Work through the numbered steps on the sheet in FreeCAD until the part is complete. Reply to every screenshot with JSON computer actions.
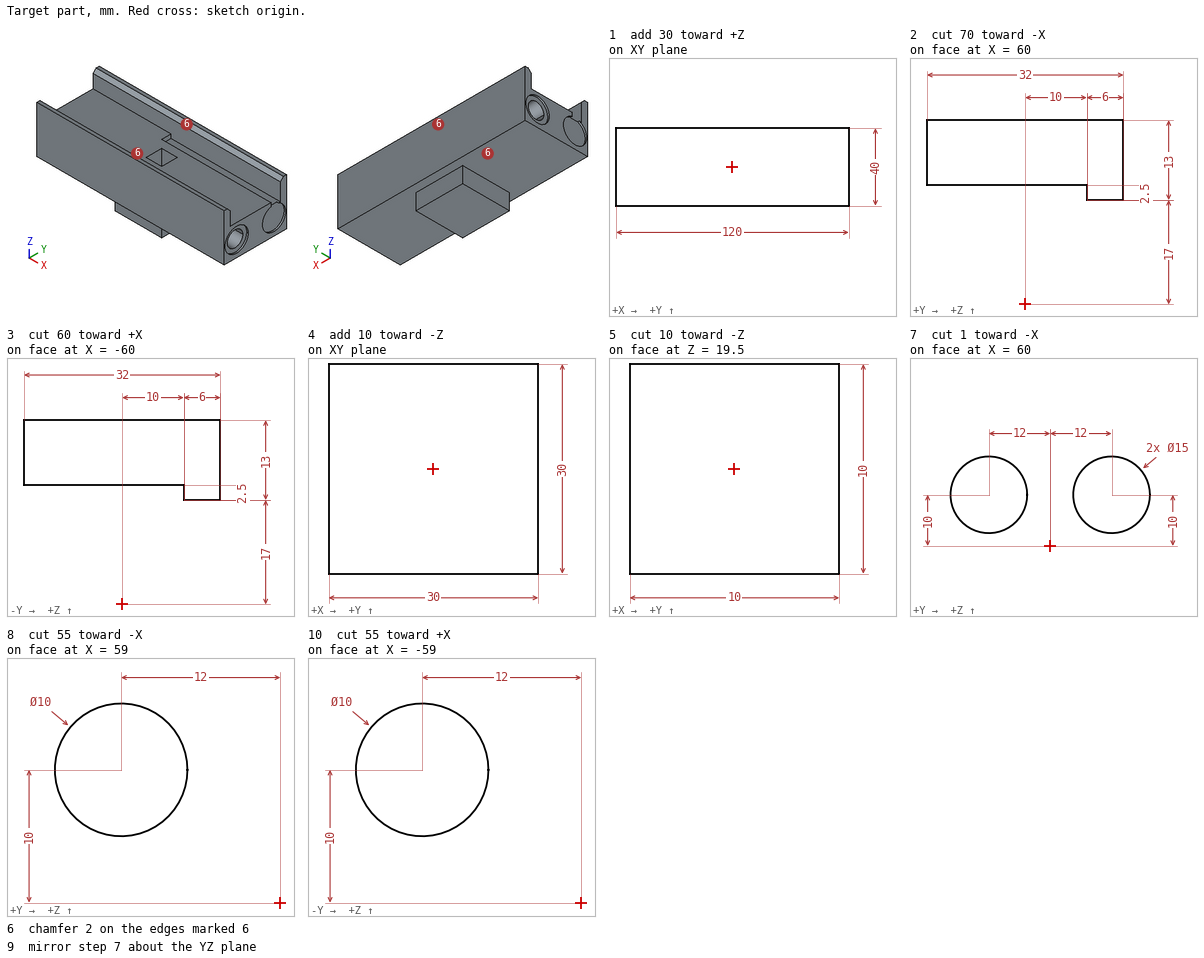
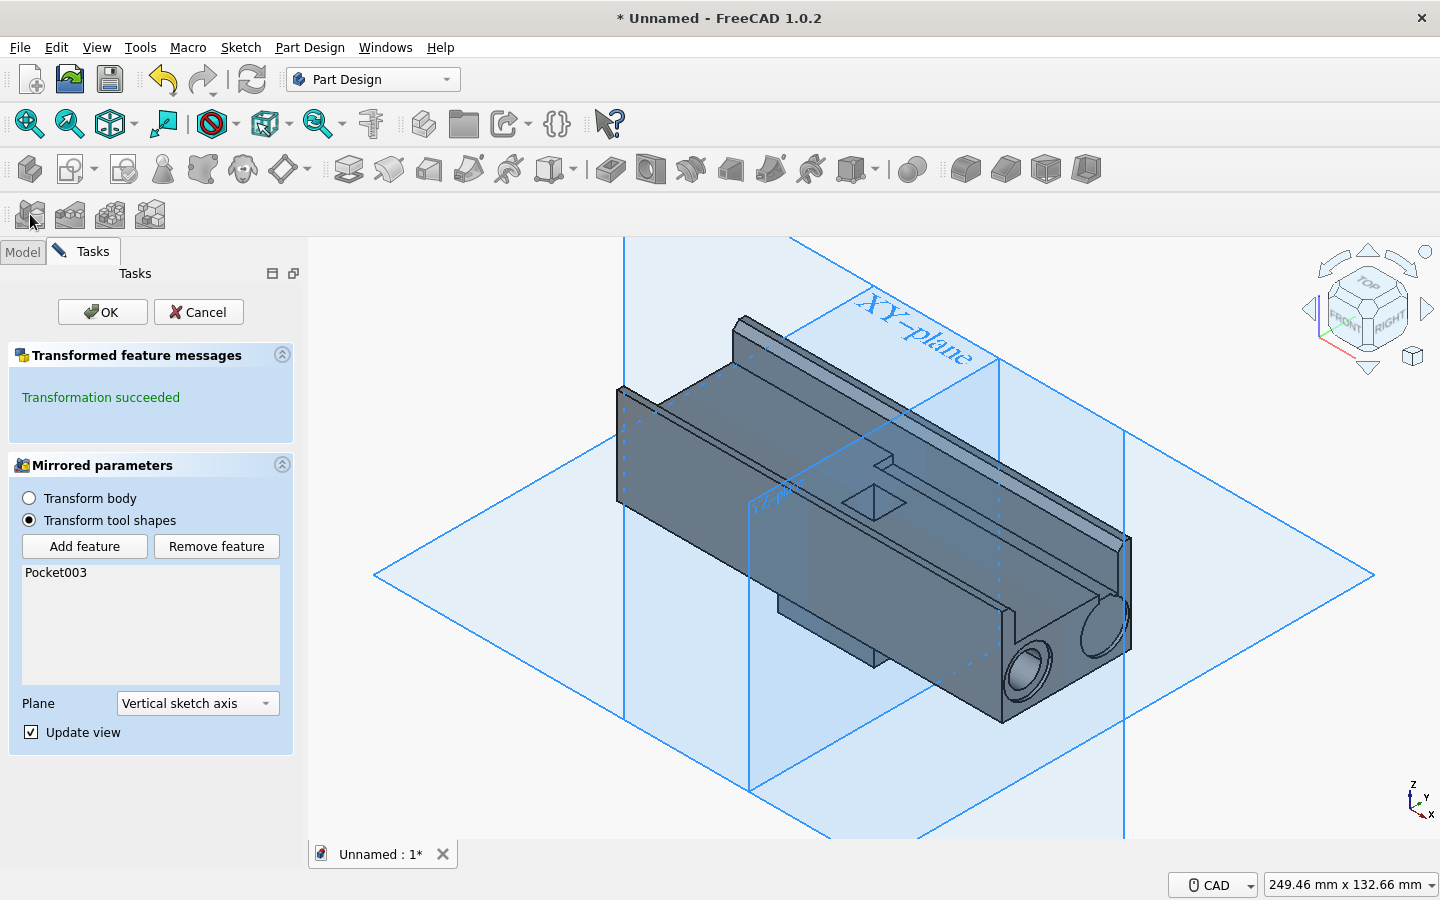
{"action": "left_click", "coordinate": [198, 704]}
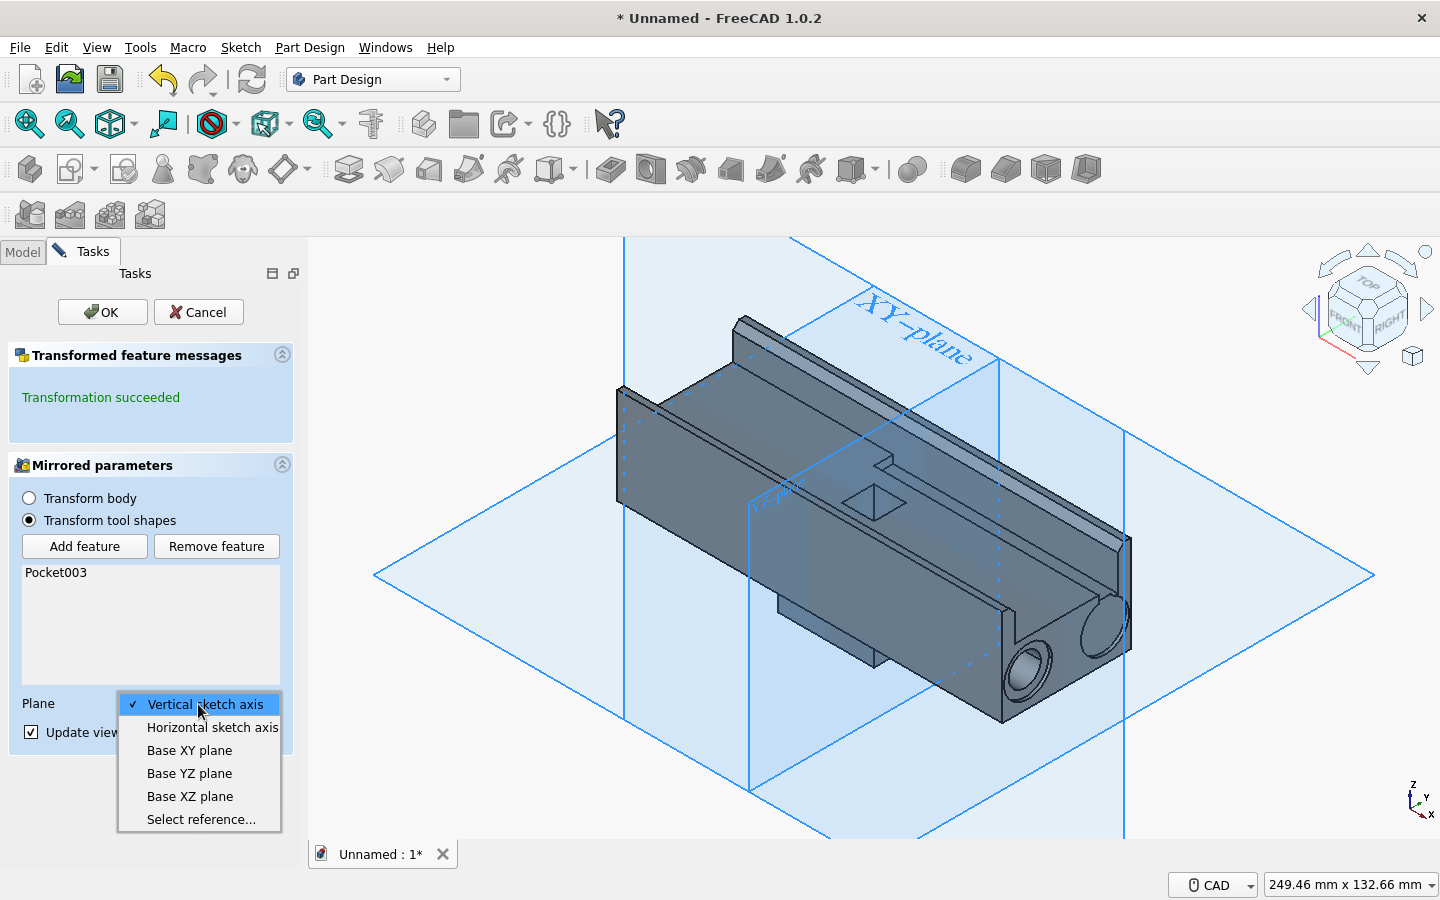
{"action": "left_click", "coordinate": [198, 774]}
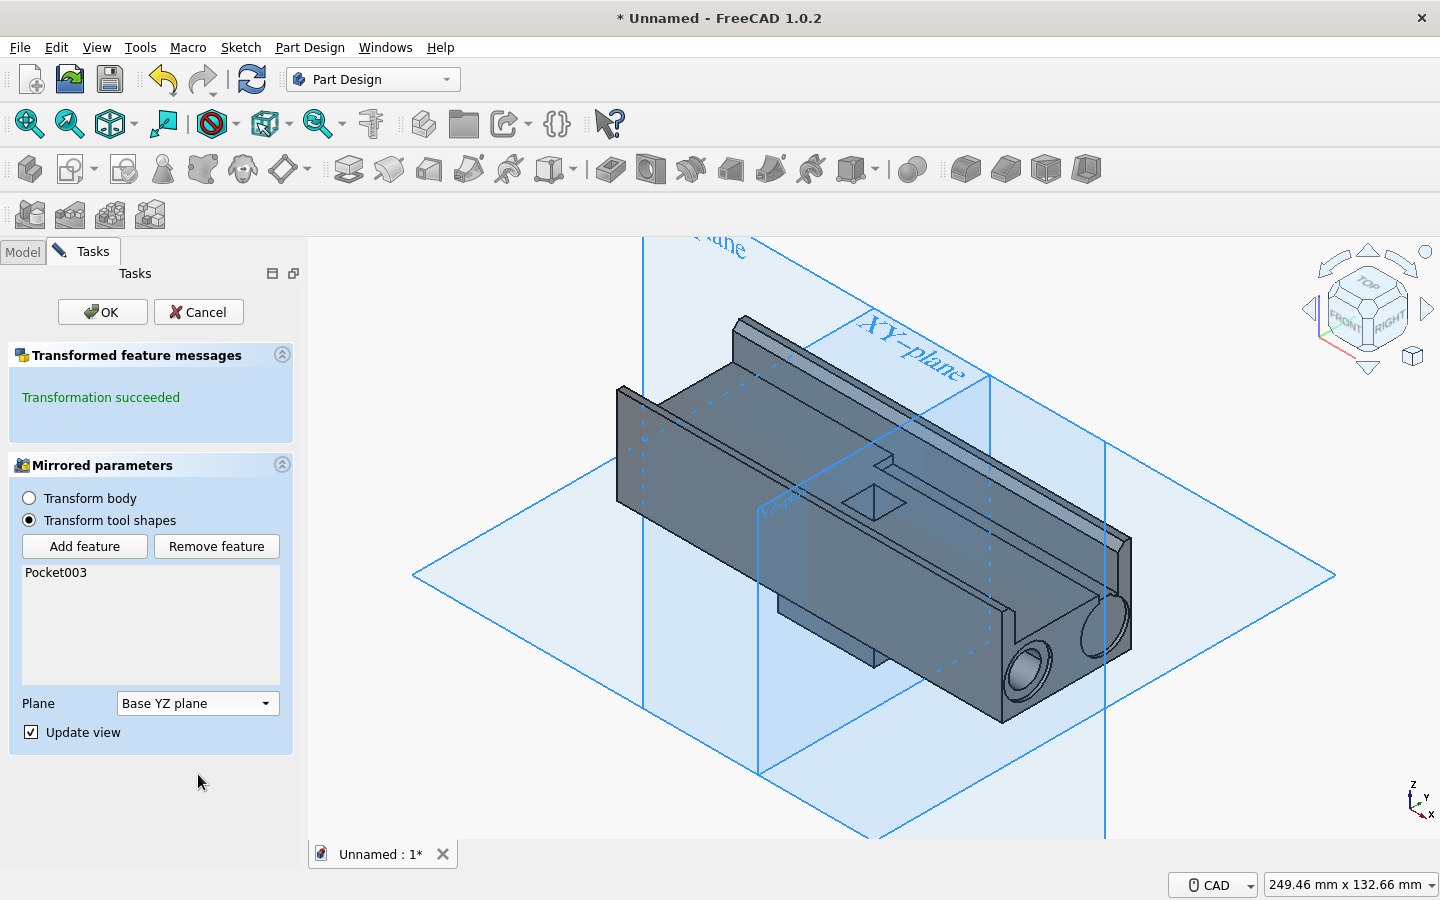
{"action": "left_click", "coordinate": [103, 312]}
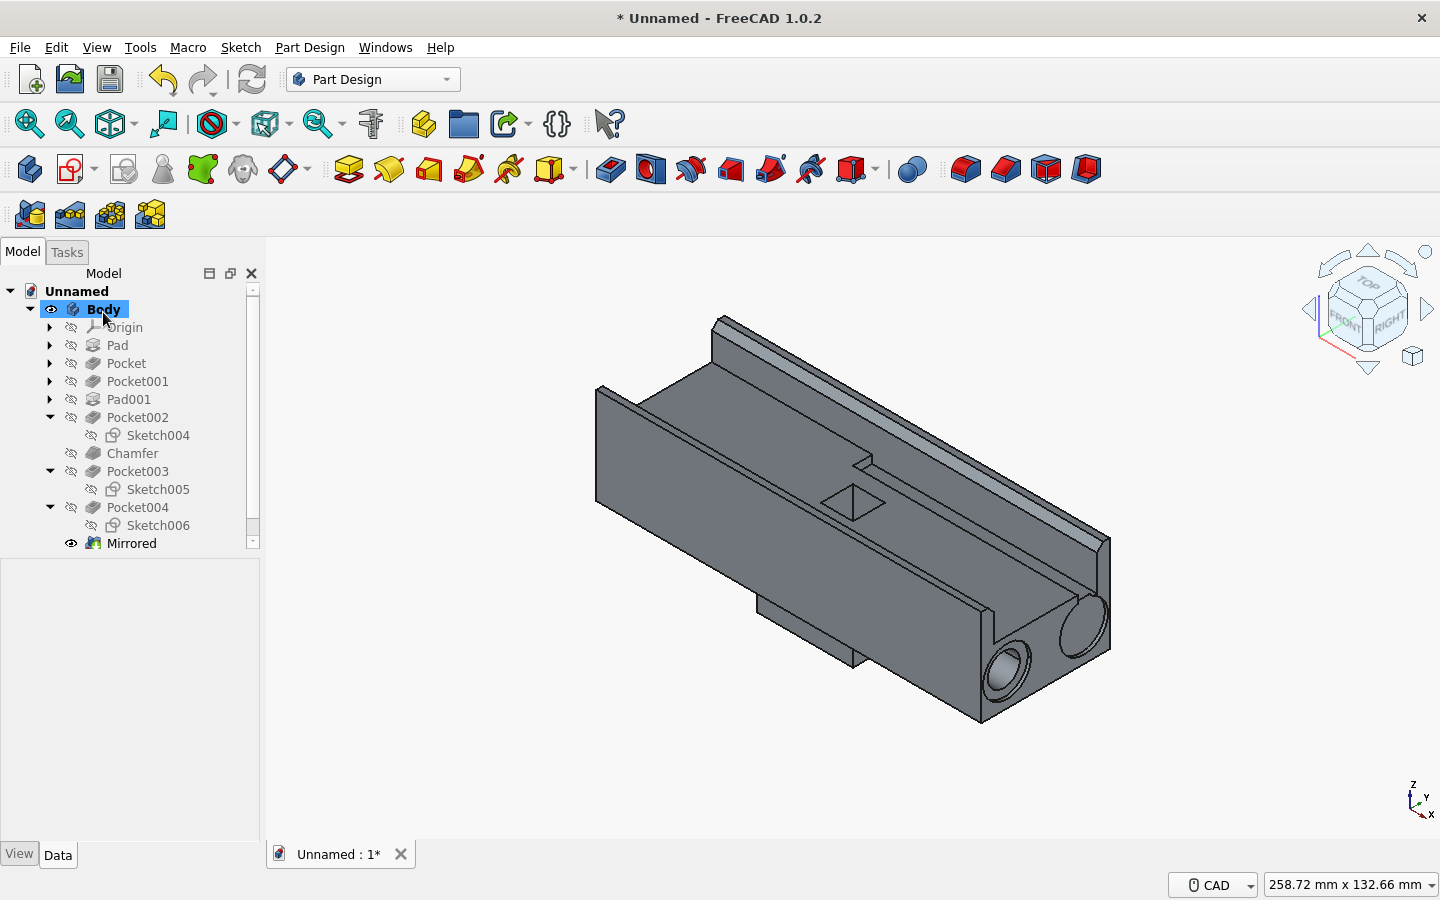
{"action": "key", "text": "6"}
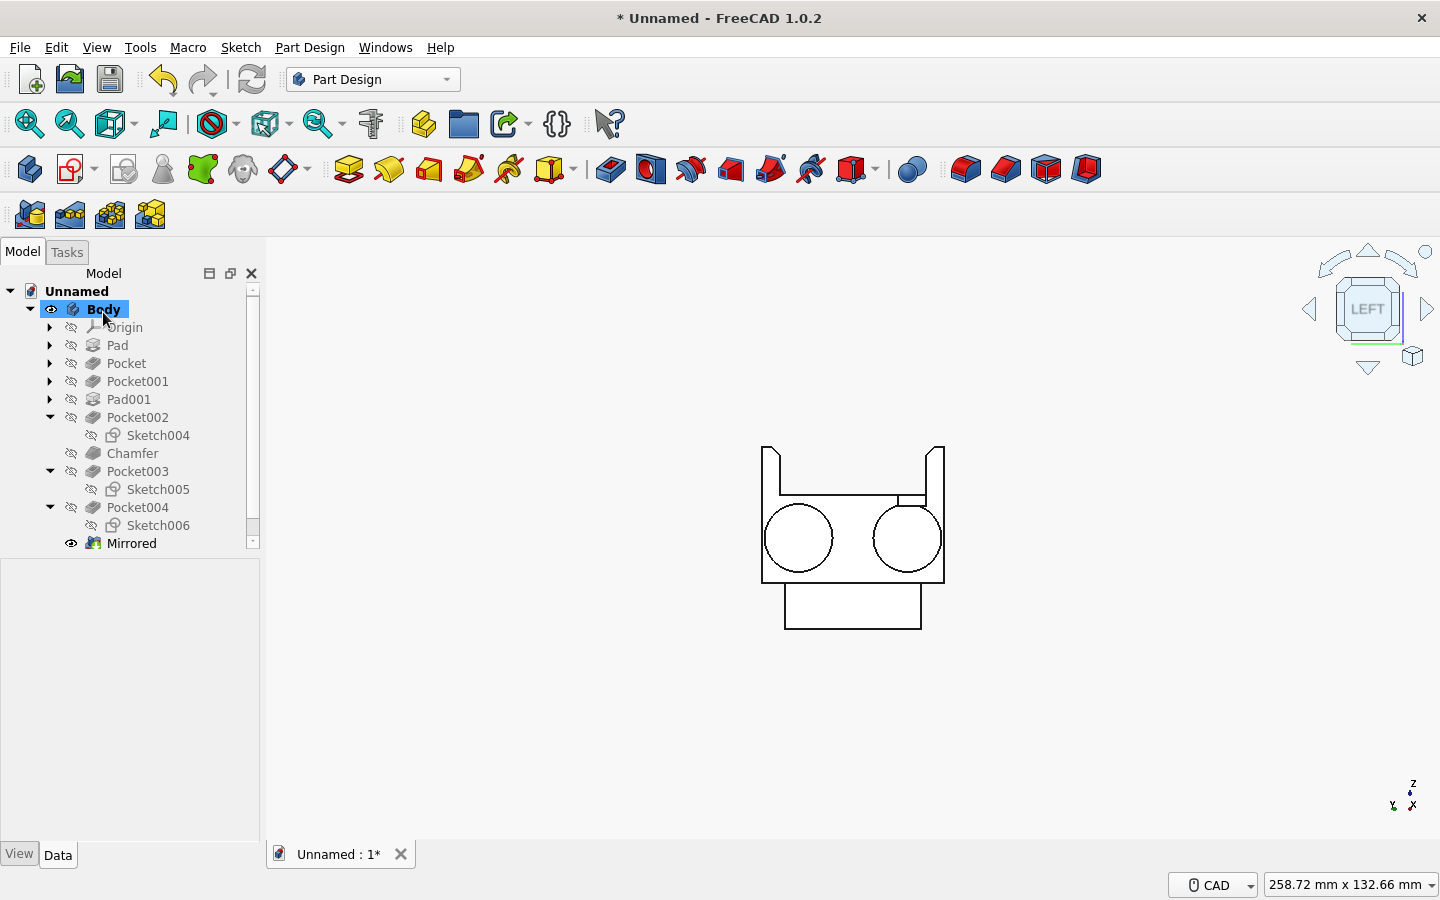
{"action": "key", "text": "v f"}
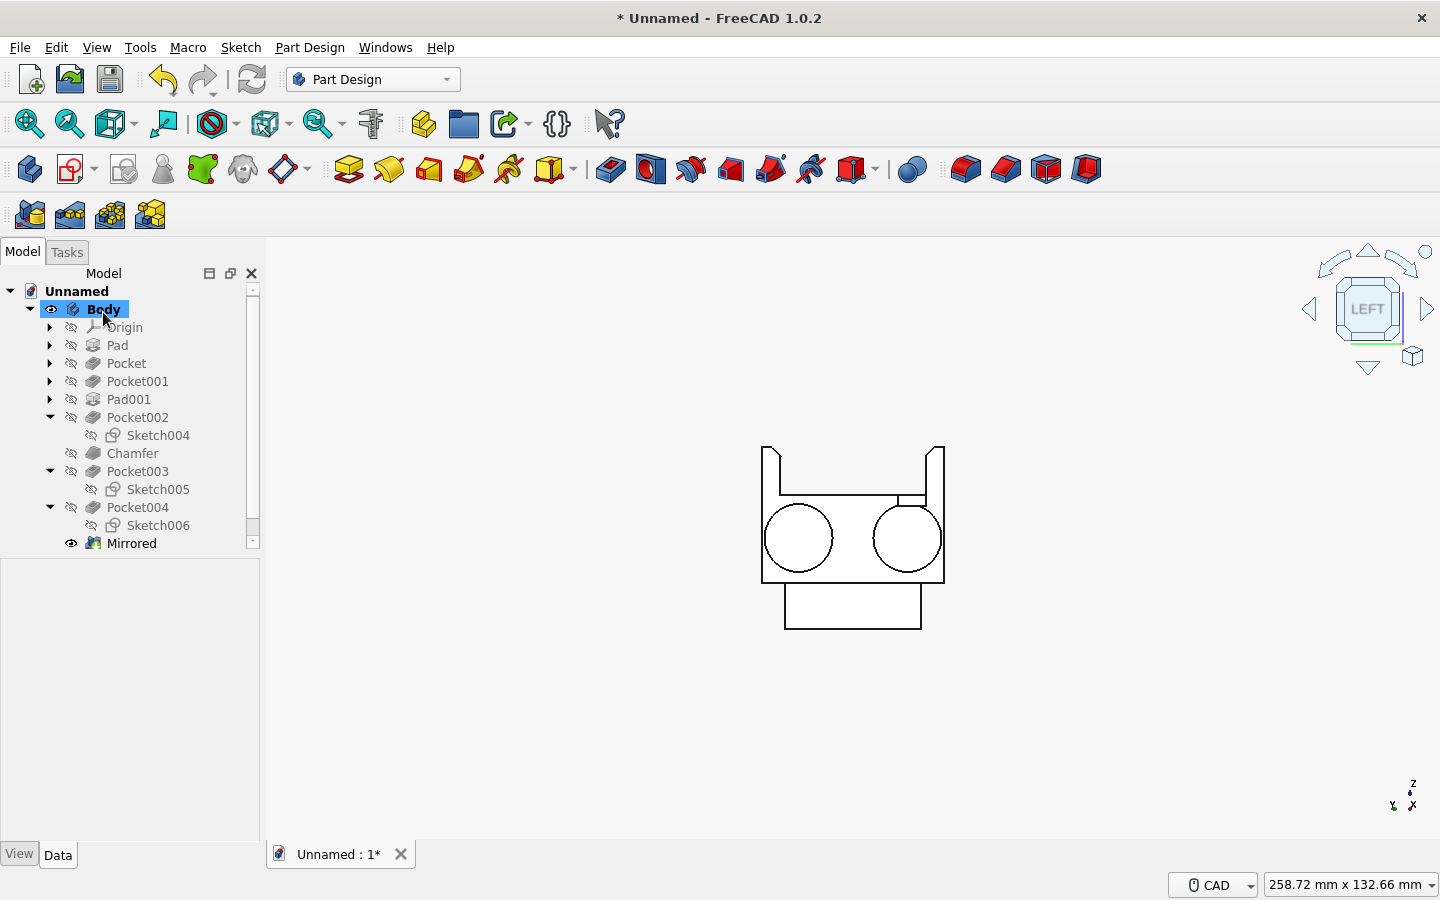
{"action": "left_click", "coordinate": [799, 537]}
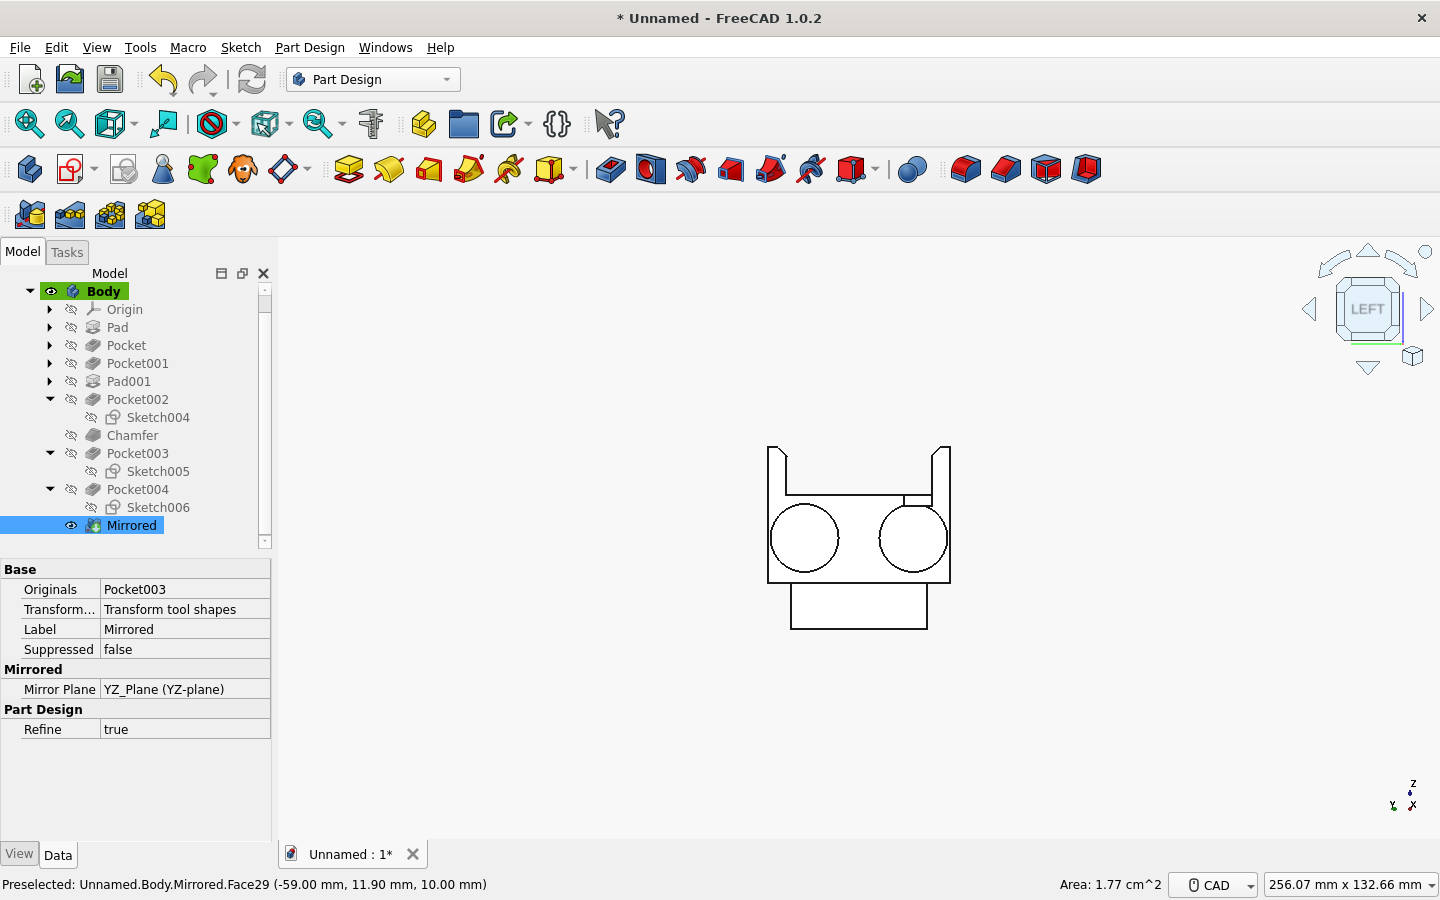
{"action": "left_click", "coordinate": [70, 170]}